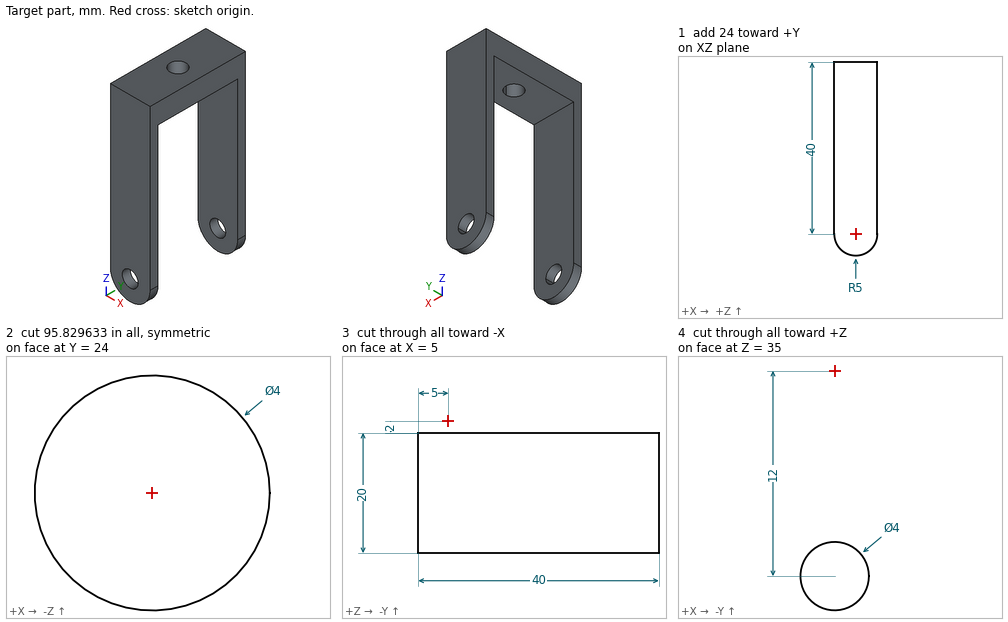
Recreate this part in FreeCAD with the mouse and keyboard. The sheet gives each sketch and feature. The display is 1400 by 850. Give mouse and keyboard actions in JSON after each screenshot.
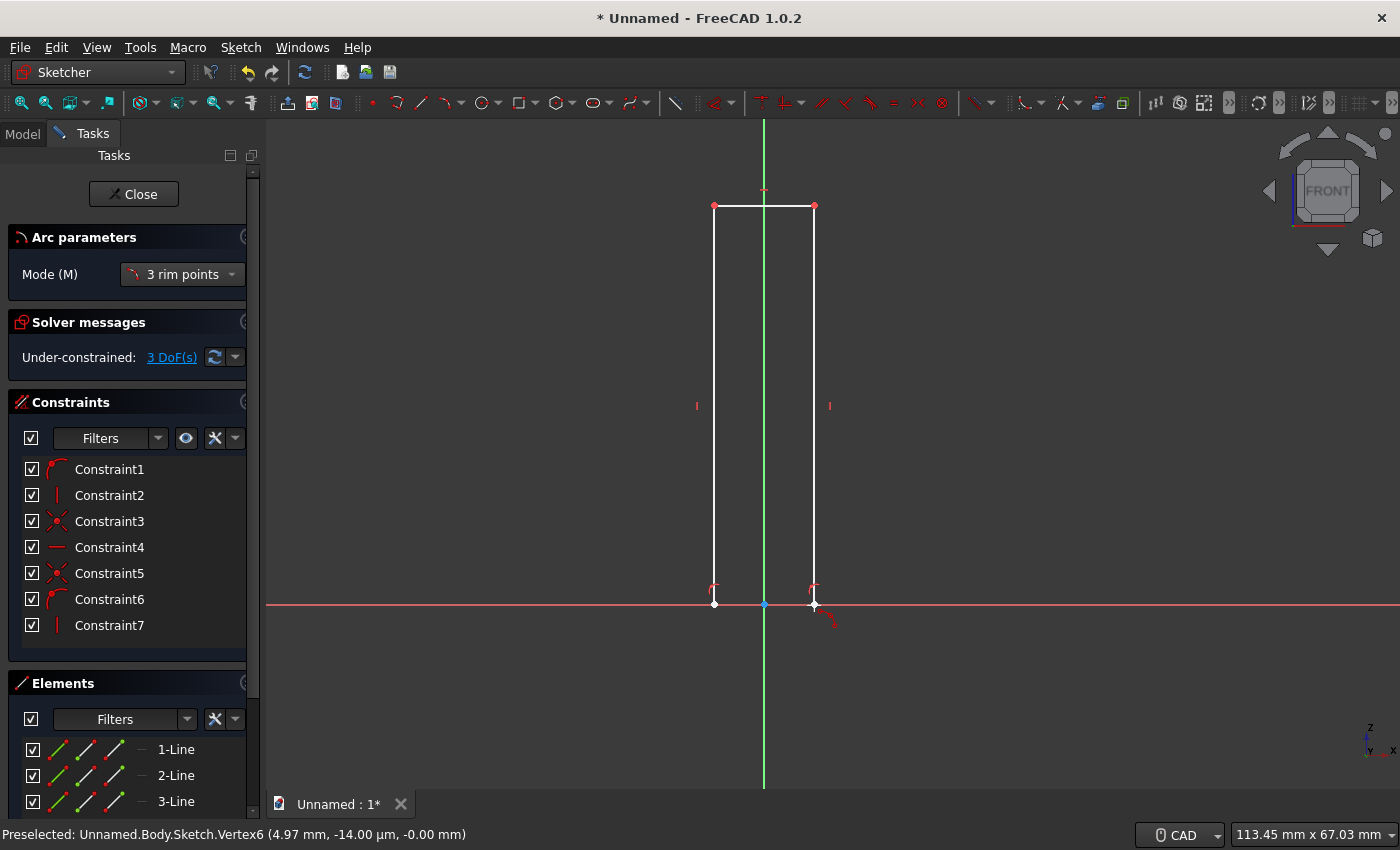
{"action": "left_click", "coordinate": [814, 605]}
{"action": "left_click", "coordinate": [714, 605]}
{"action": "left_click", "coordinate": [749, 652]}
{"action": "key", "text": "Escape"}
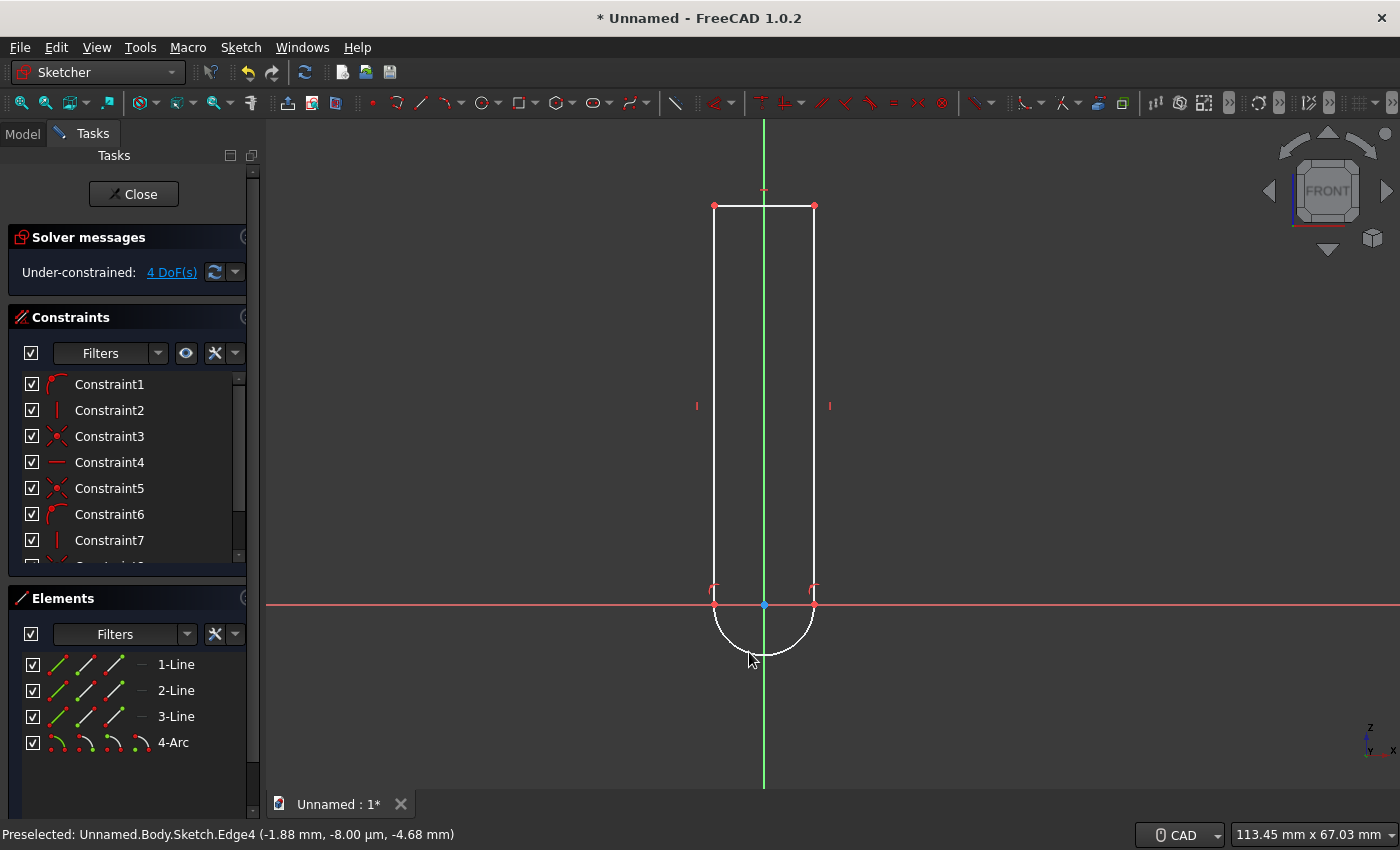
{"action": "left_click", "coordinate": [714, 485]}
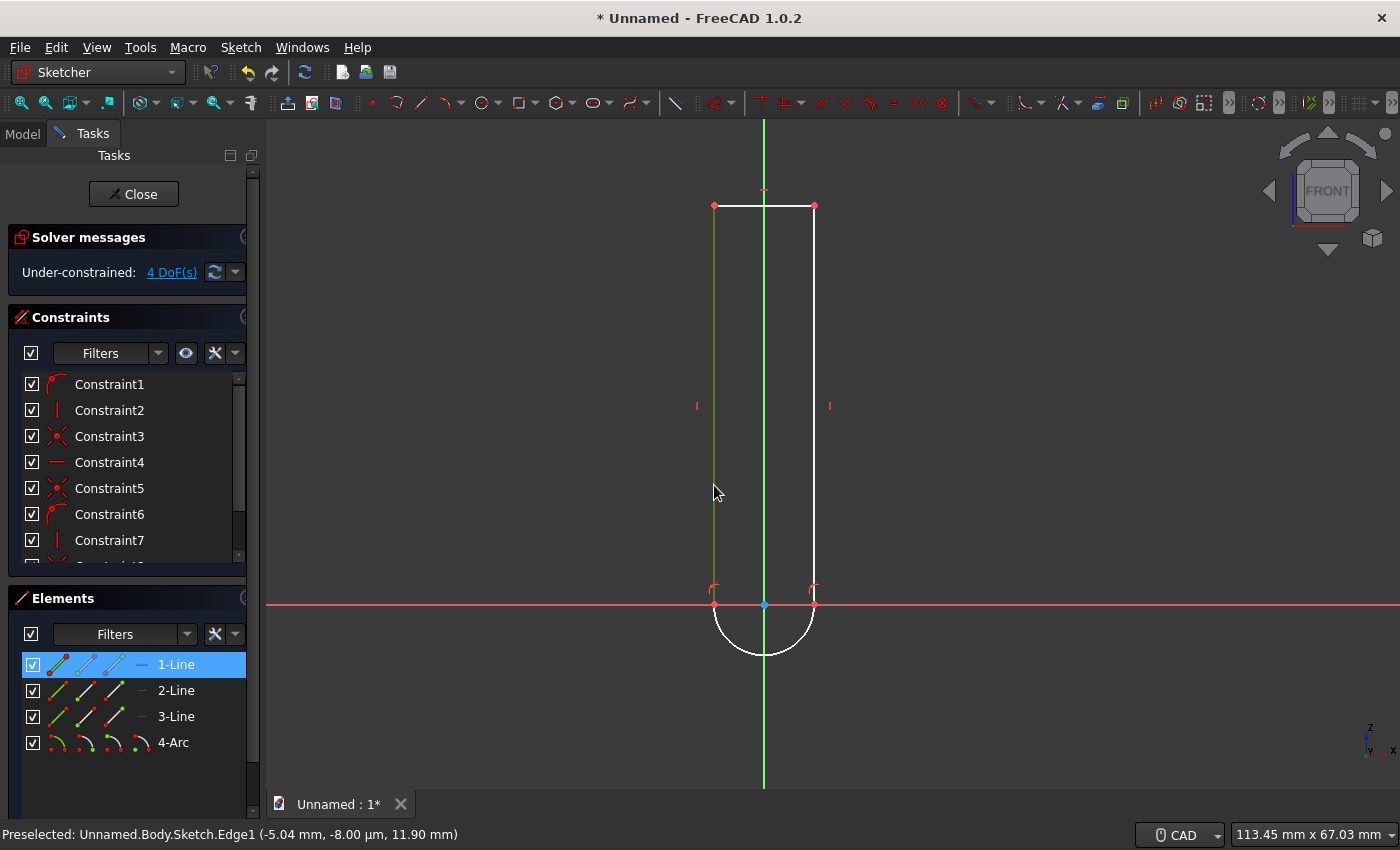
{"action": "left_click", "coordinate": [735, 646]}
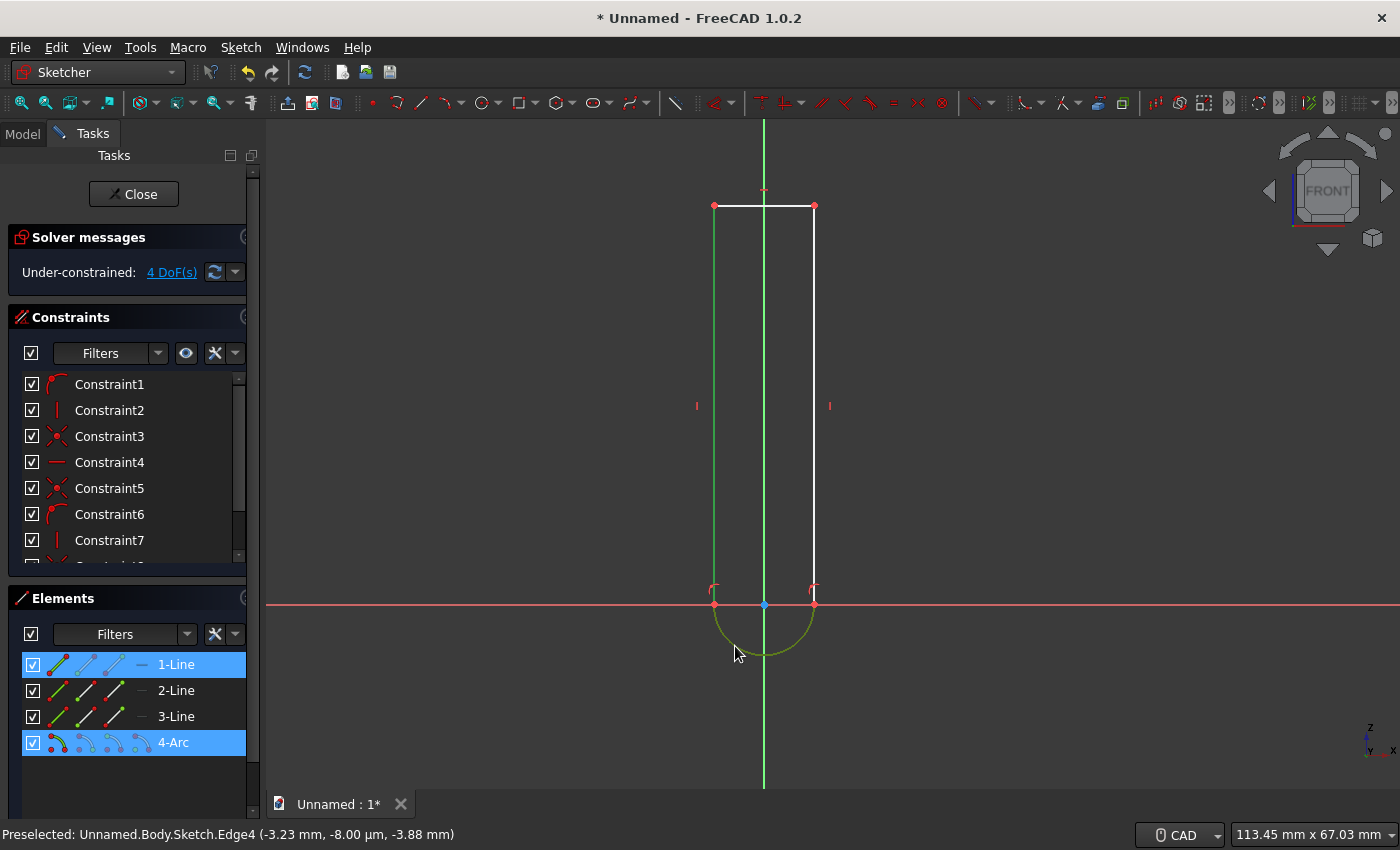
{"action": "key", "text": "t"}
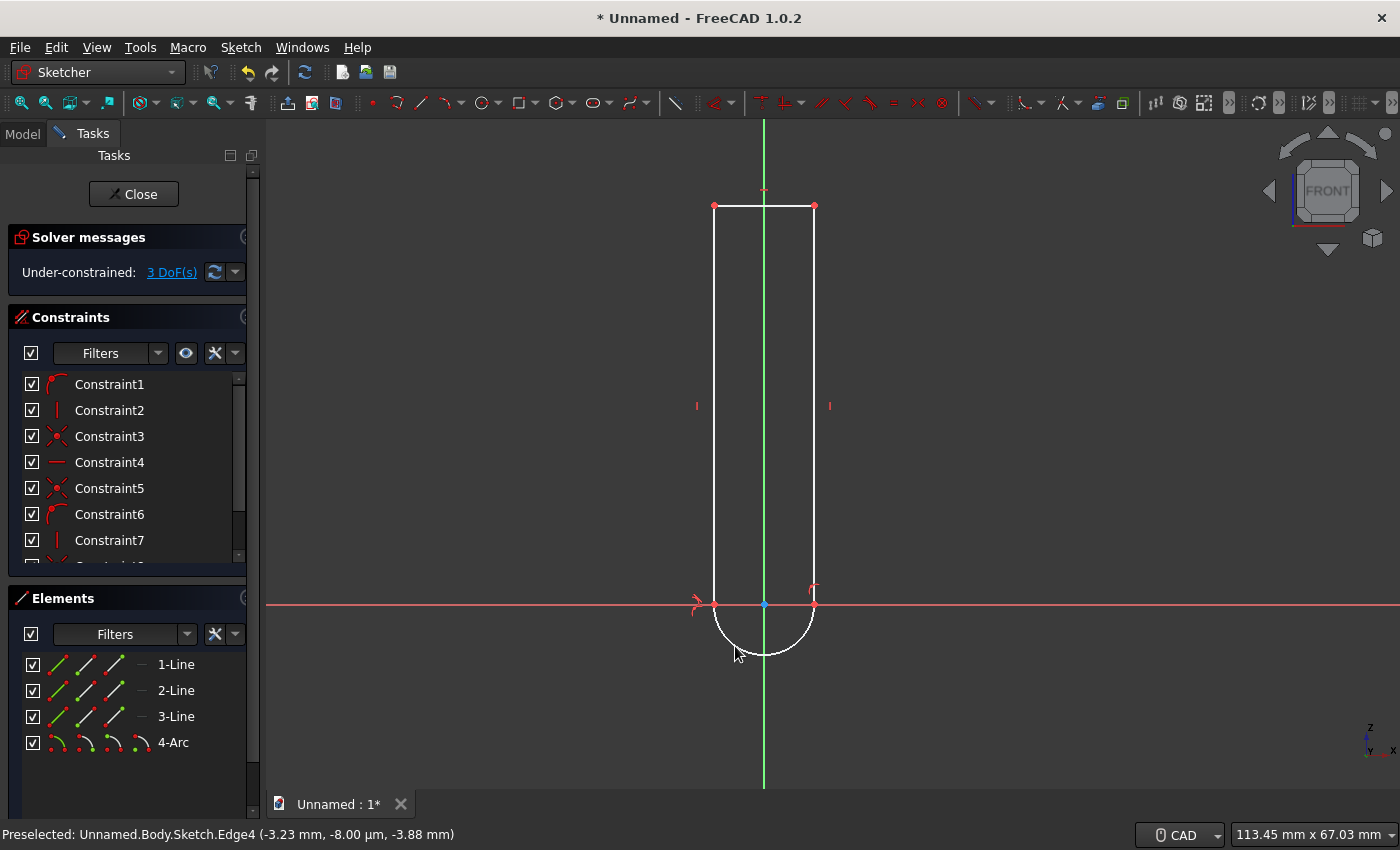
{"action": "left_click", "coordinate": [764, 605]}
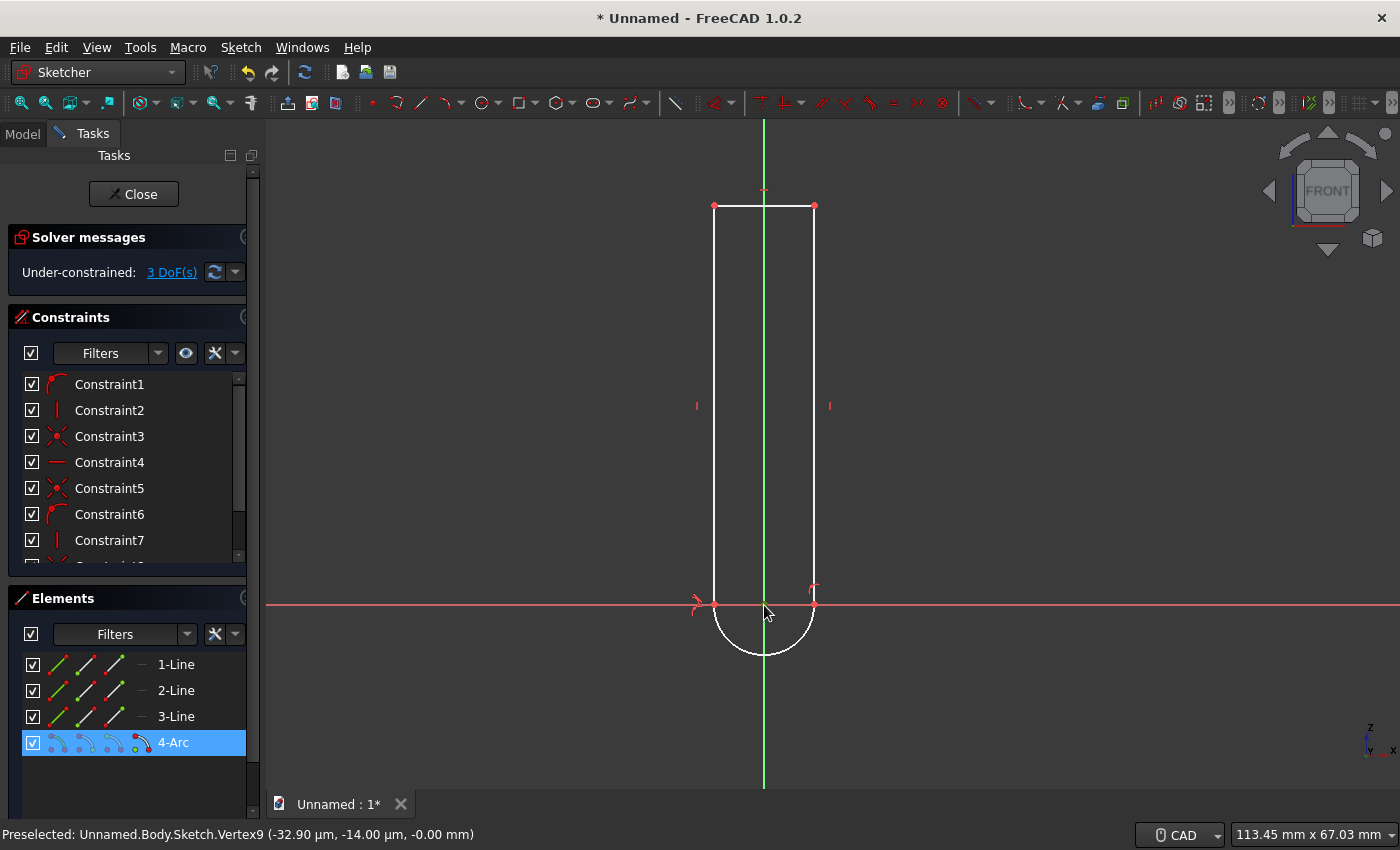
{"action": "left_click", "coordinate": [764, 717]}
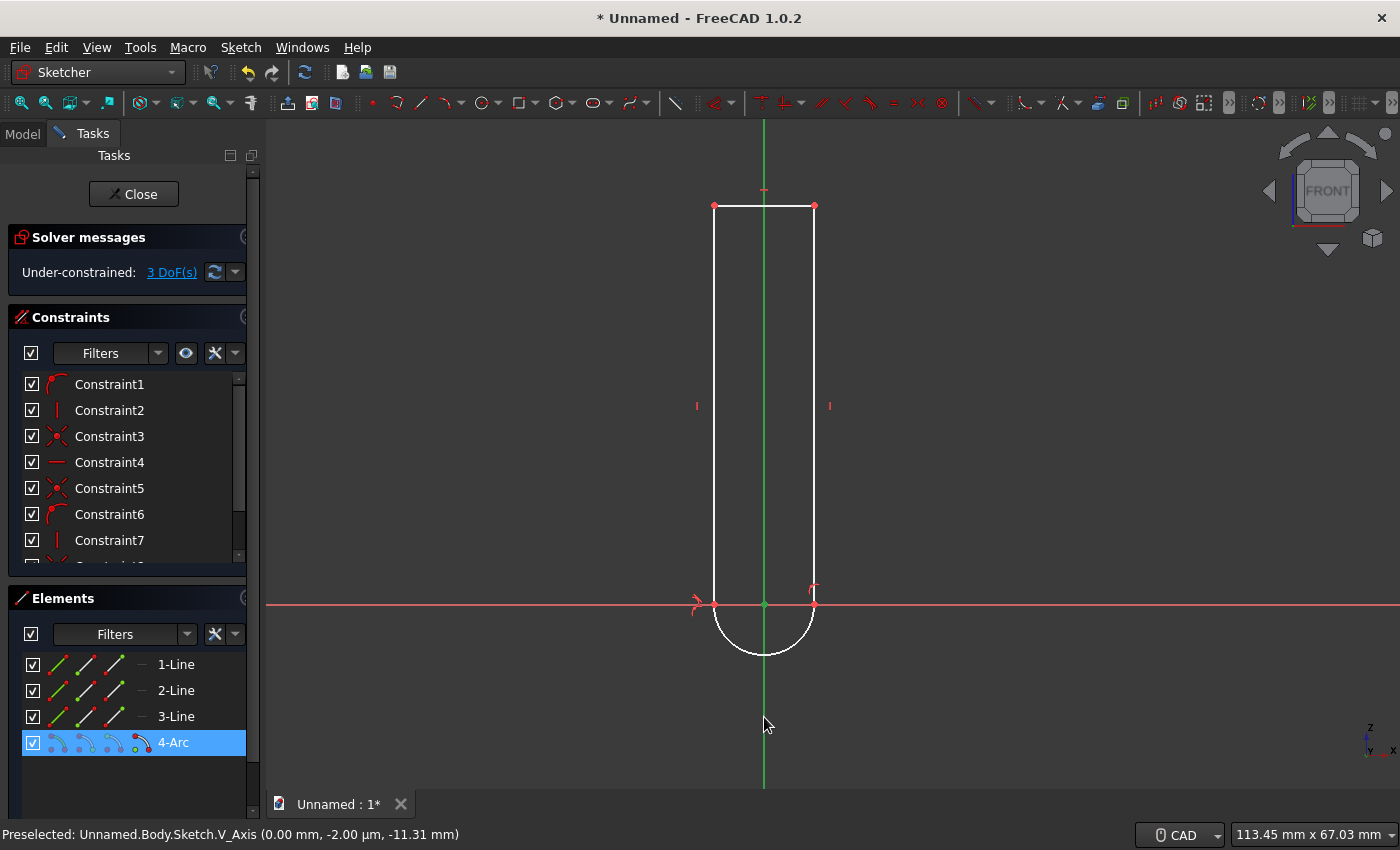
{"action": "key", "text": "c"}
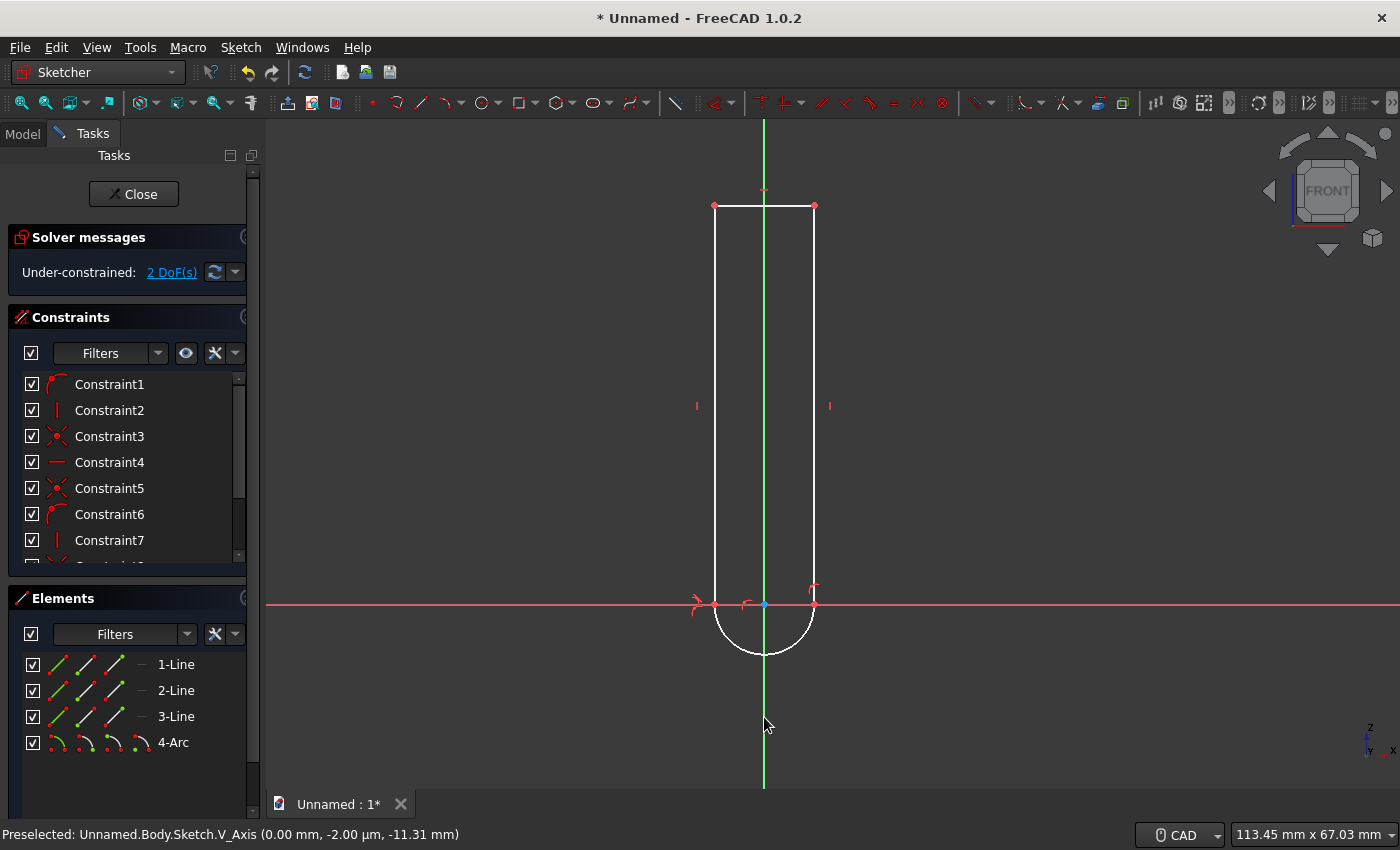
{"action": "left_click", "coordinate": [735, 645]}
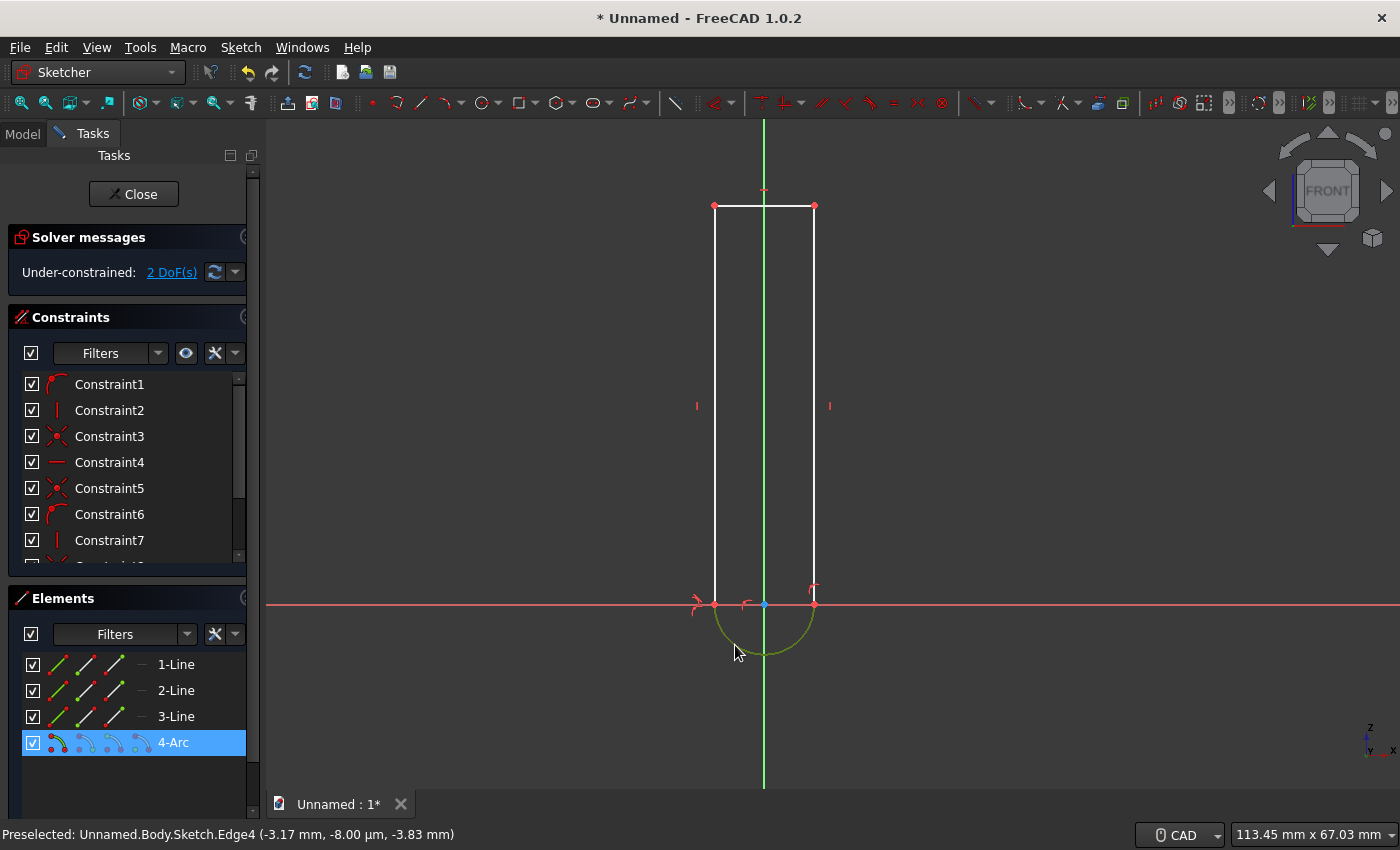
{"action": "key", "text": "k r"}